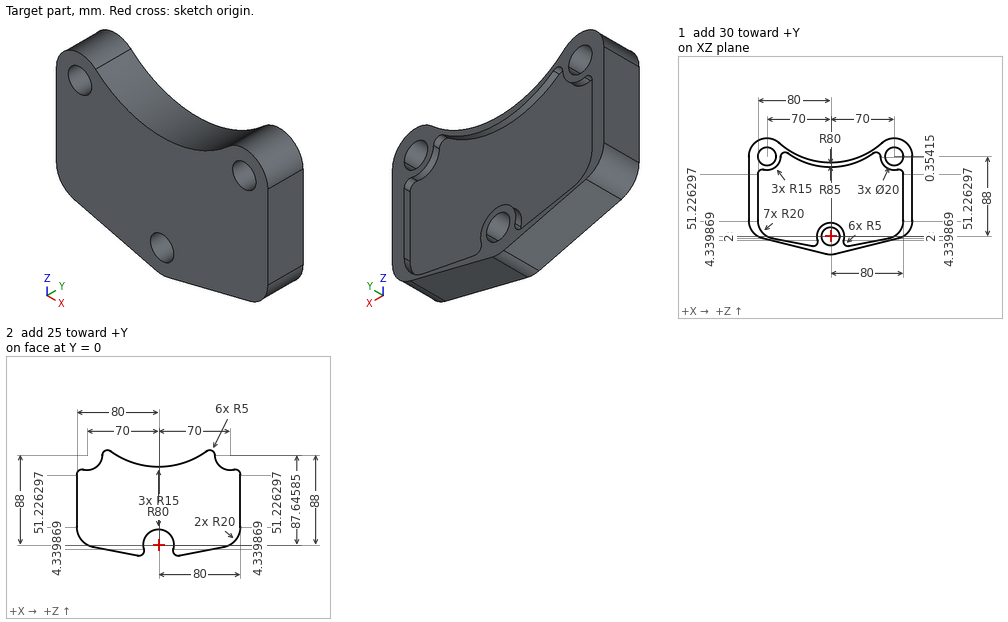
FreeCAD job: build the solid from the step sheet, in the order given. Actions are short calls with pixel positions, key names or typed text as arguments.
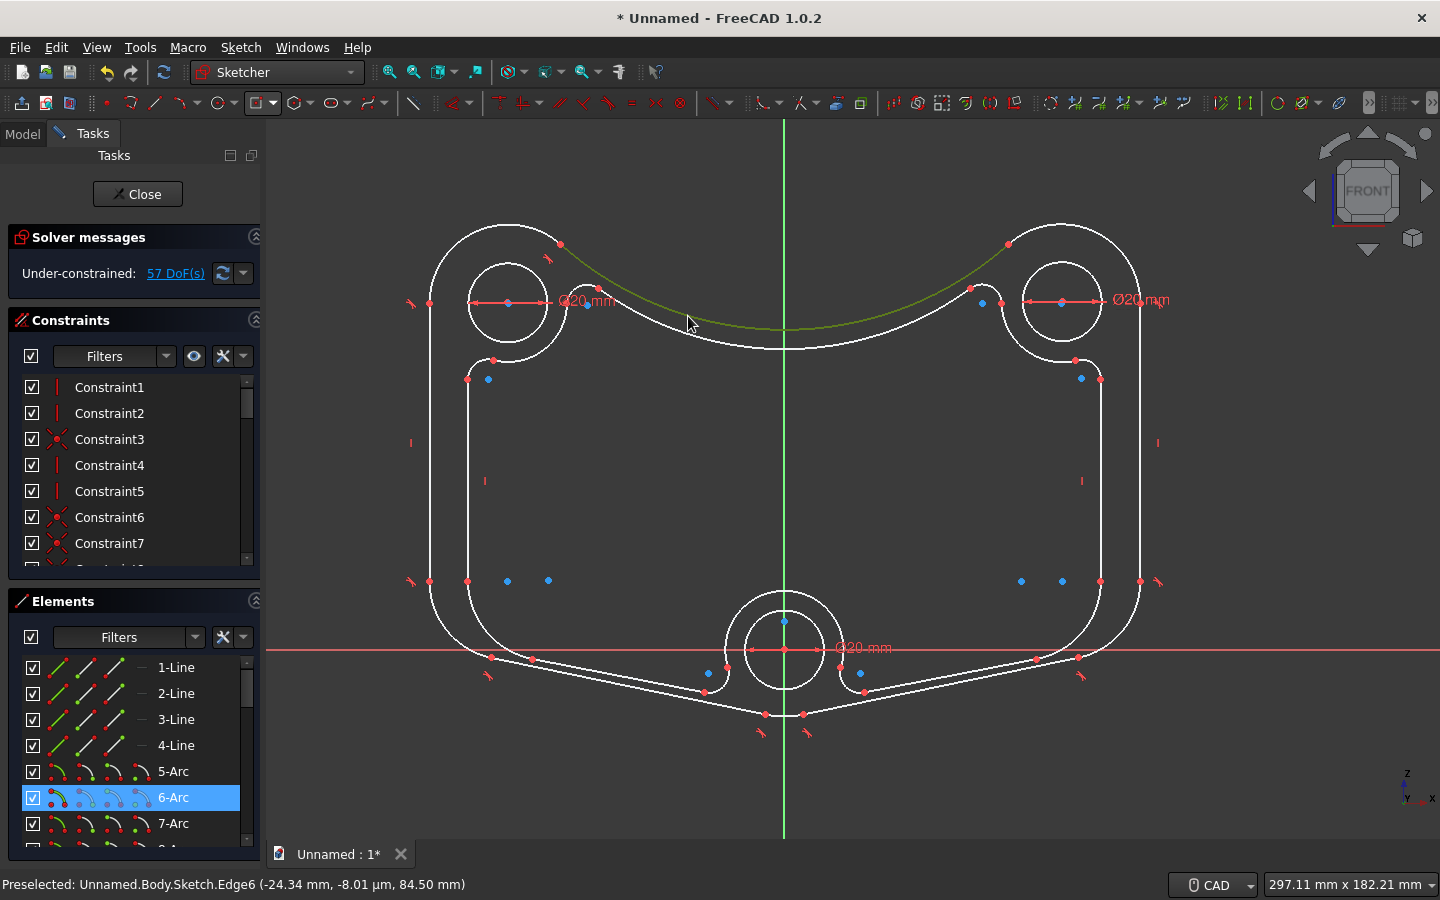
click(1122, 253)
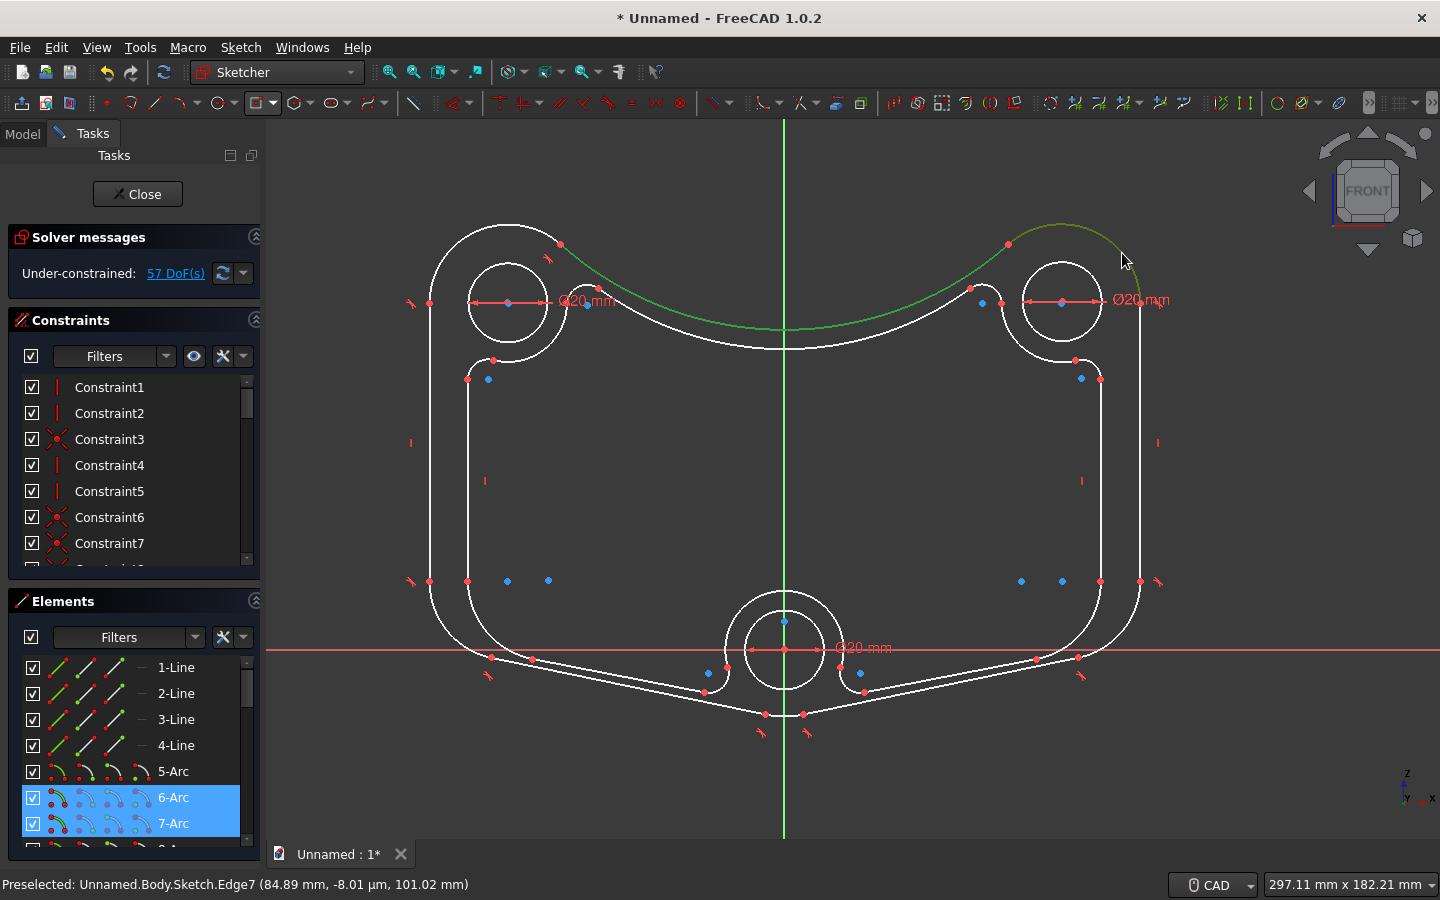
click(608, 104)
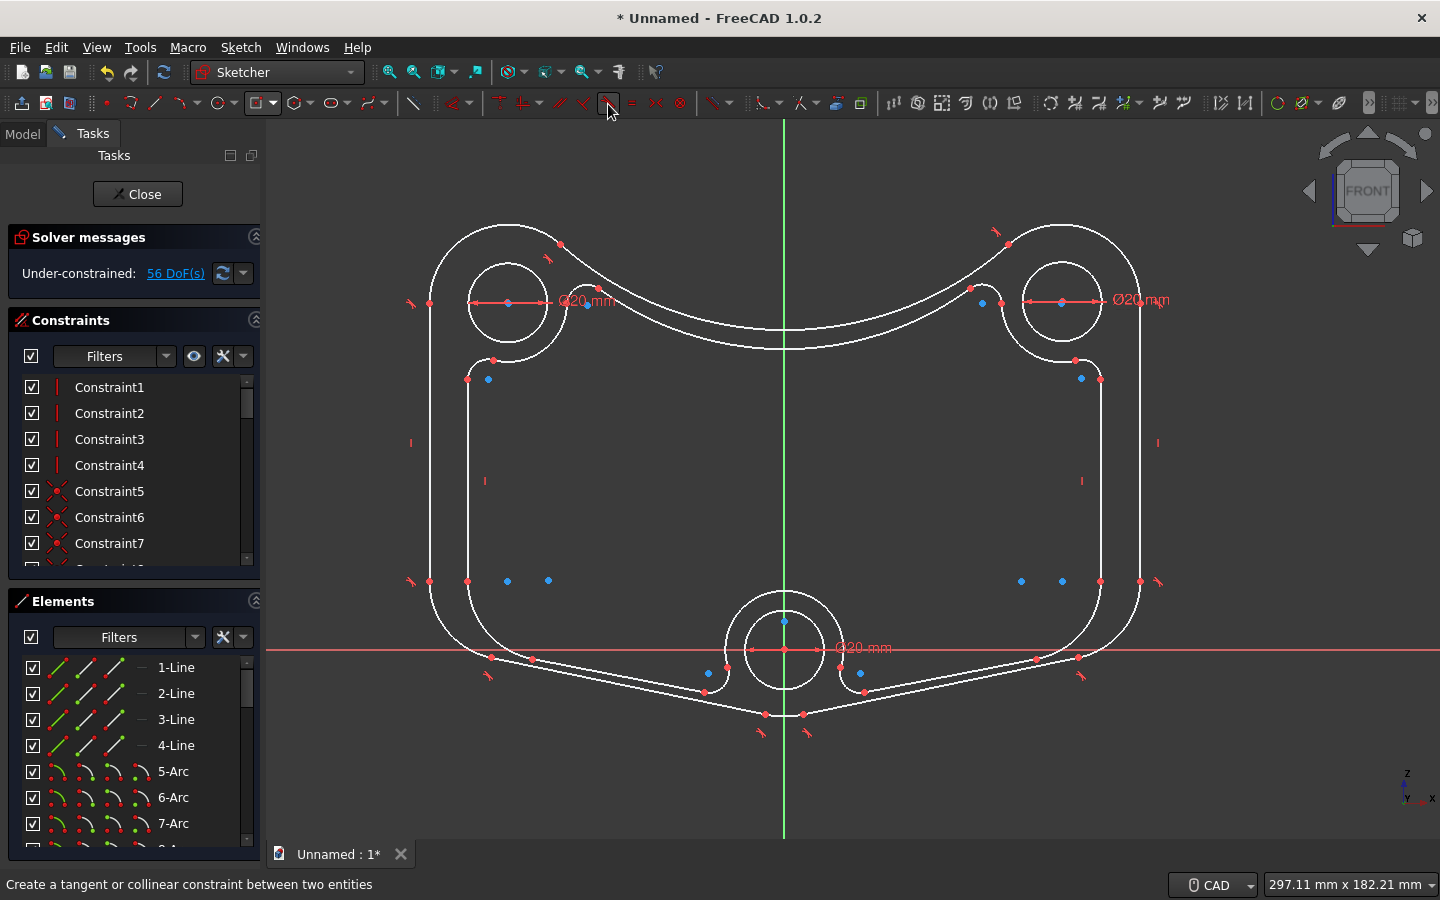
click(468, 440)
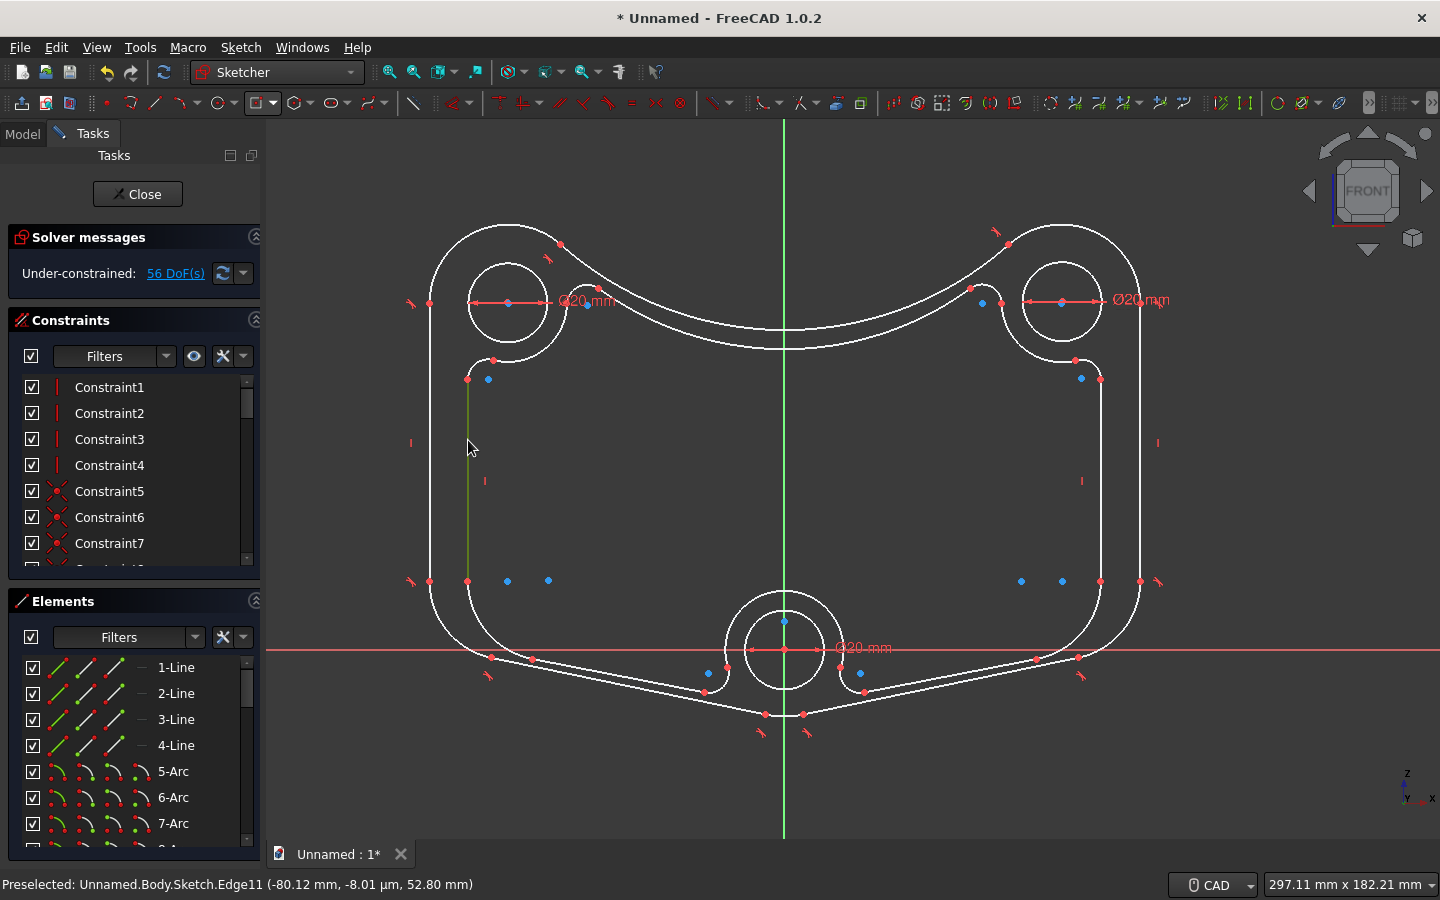
click(475, 613)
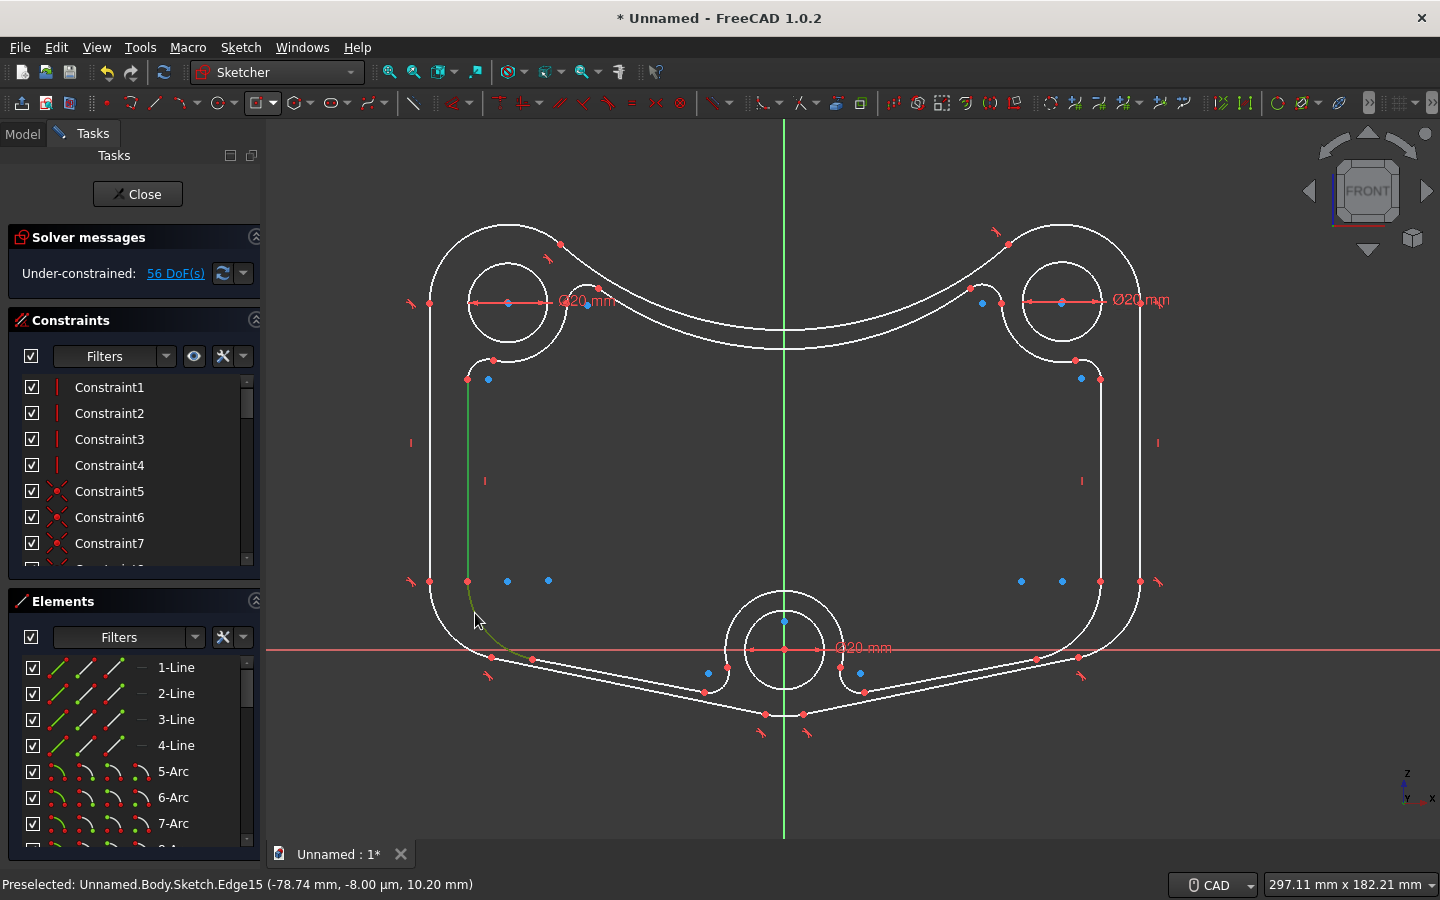
click(608, 104)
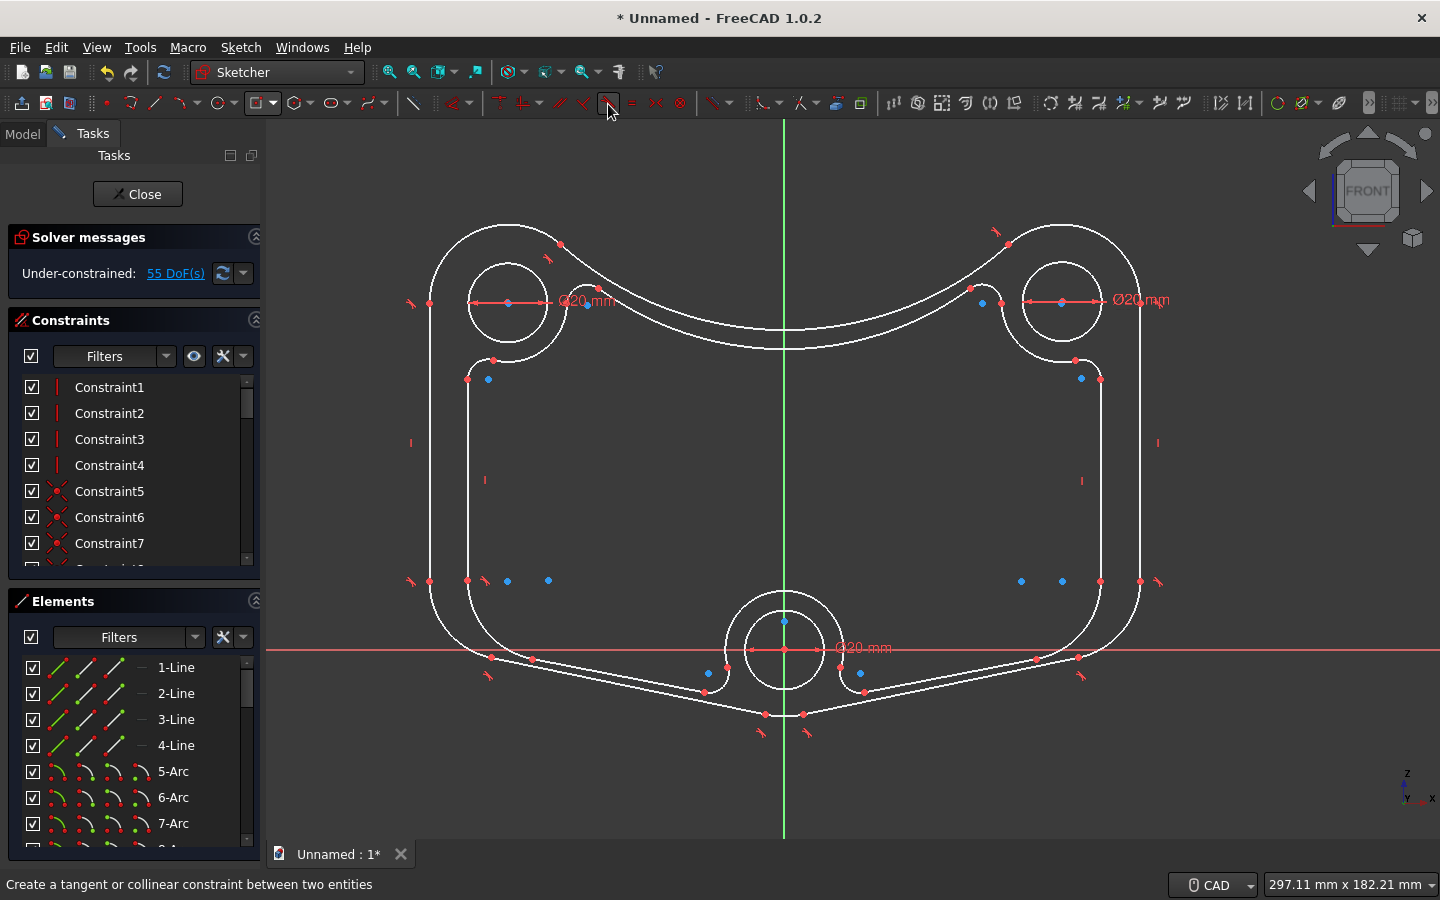
click(468, 440)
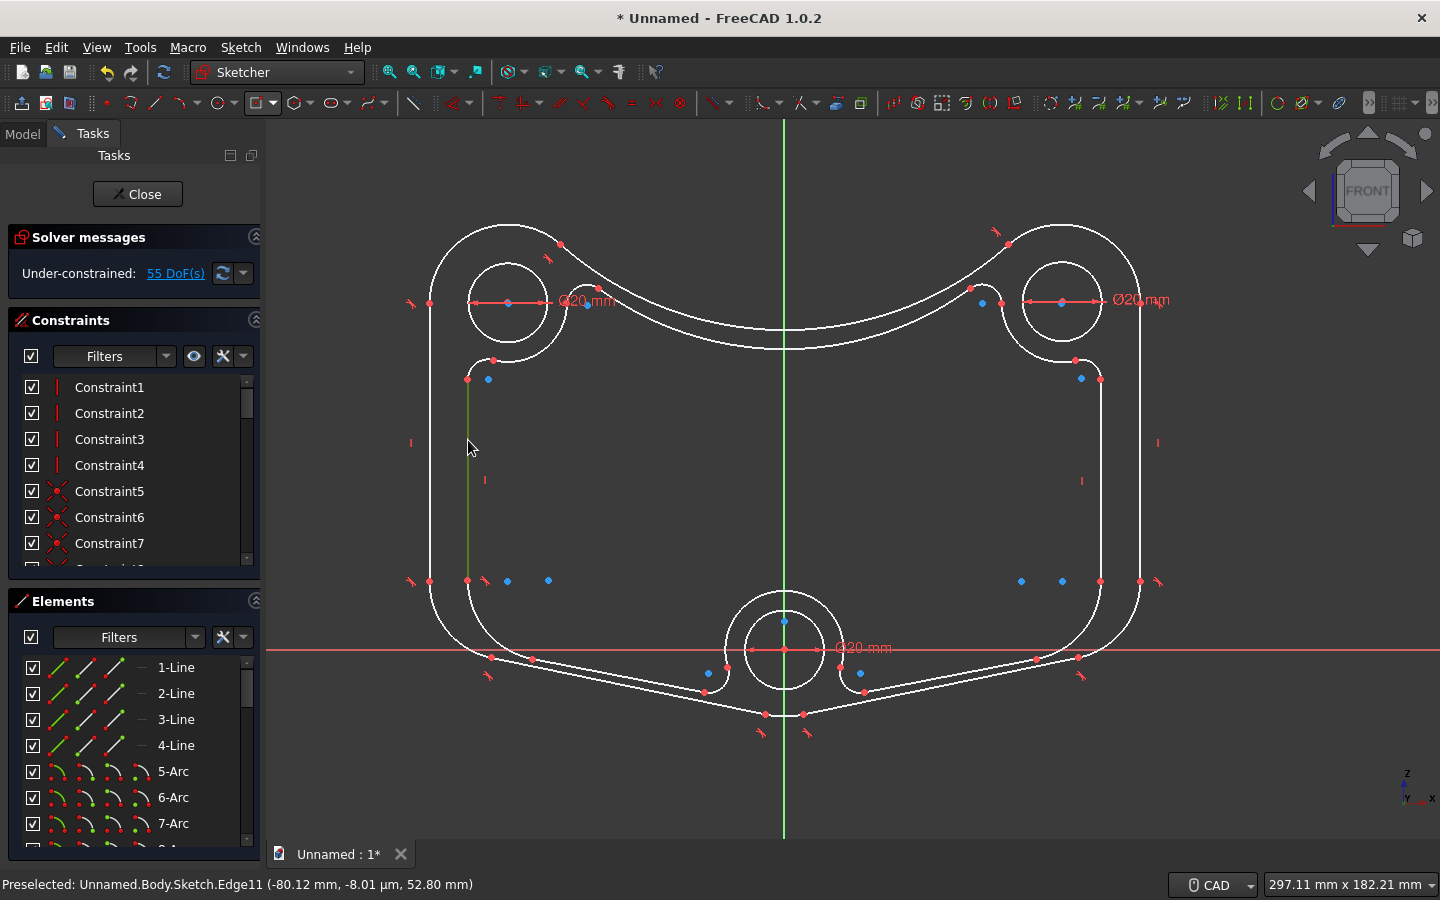
scroll(482, 360, up, 2)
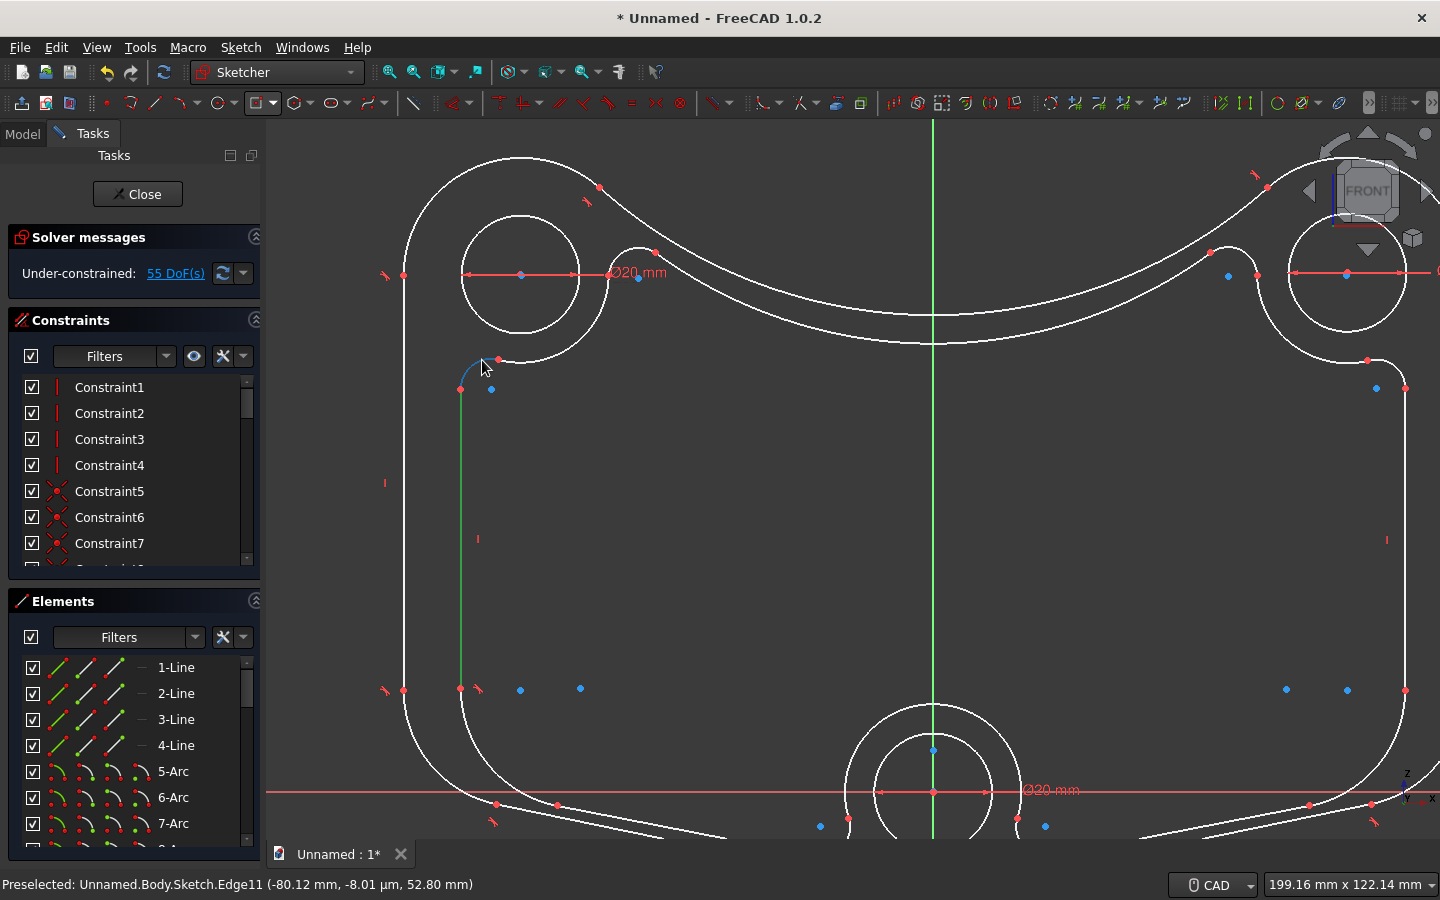
click(482, 360)